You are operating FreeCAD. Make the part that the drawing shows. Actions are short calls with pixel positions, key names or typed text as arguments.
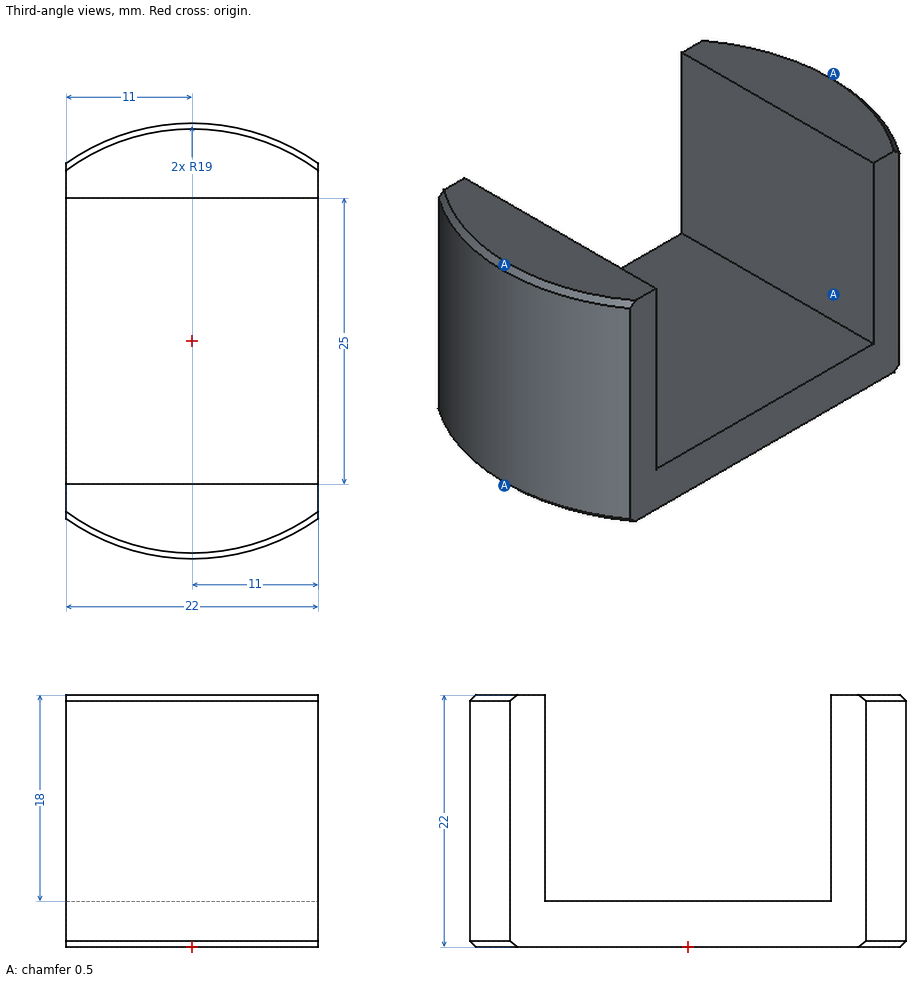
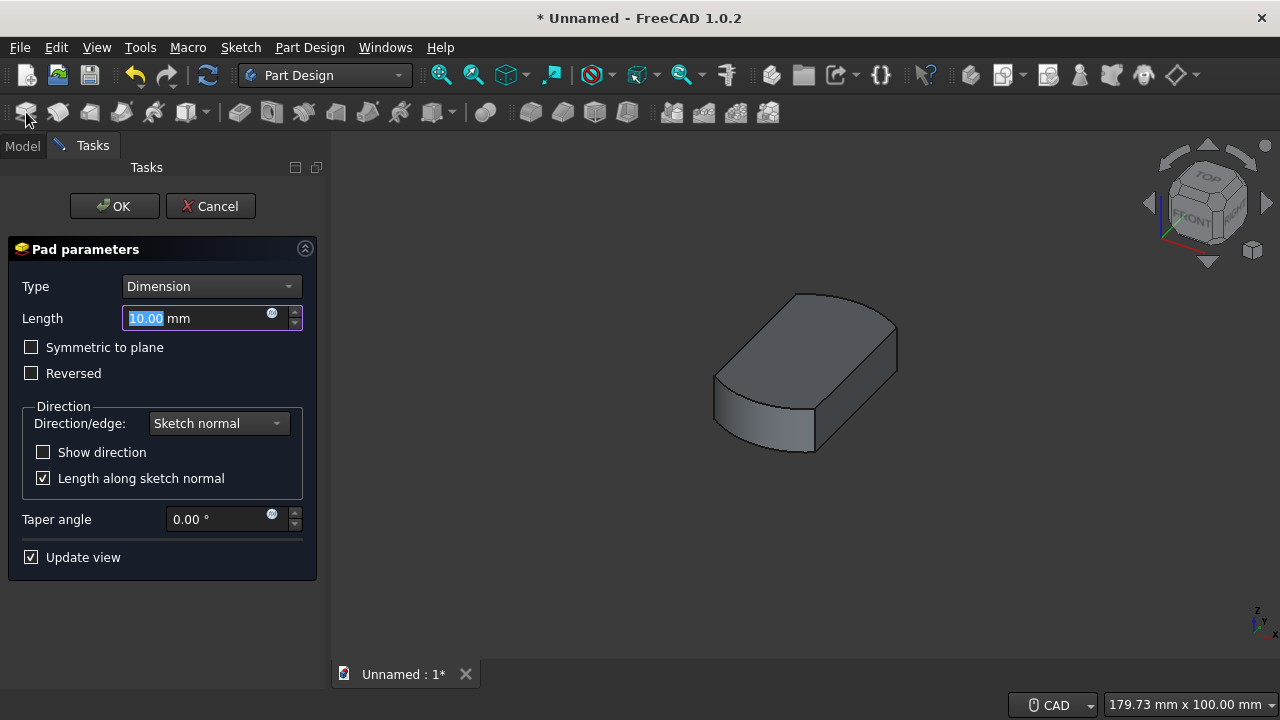
text(22)
key(Tab)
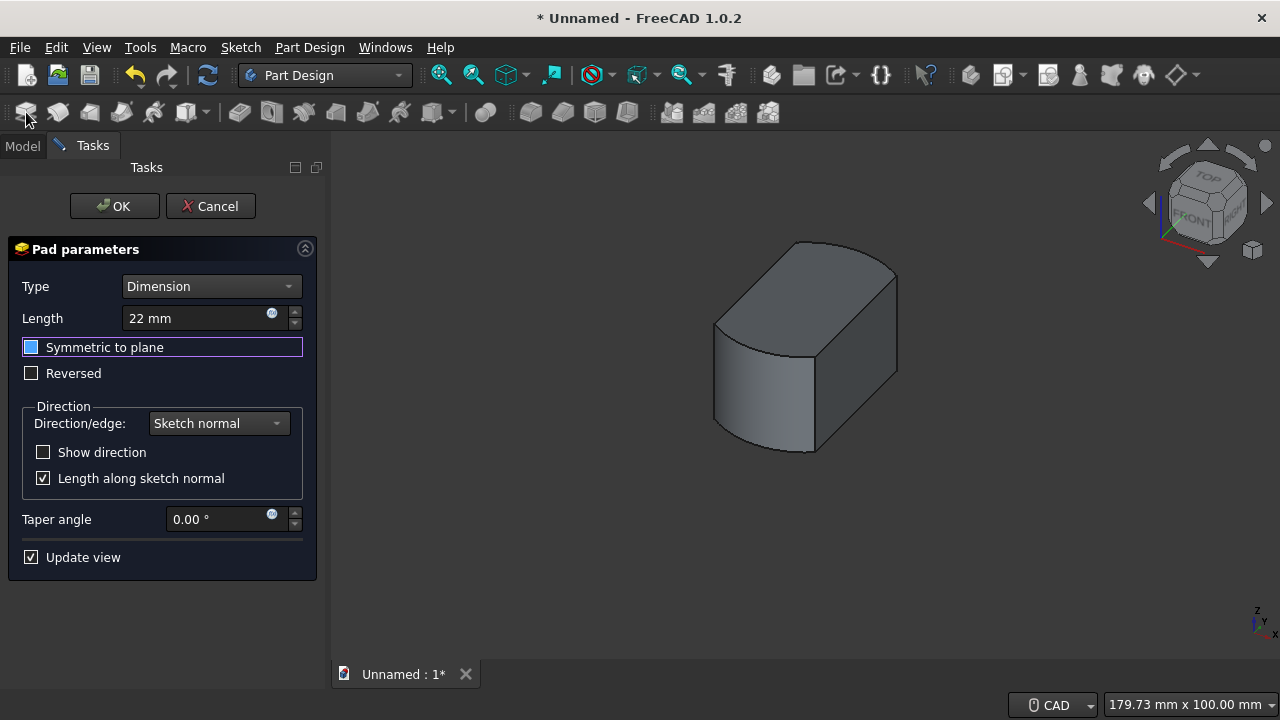
click(115, 206)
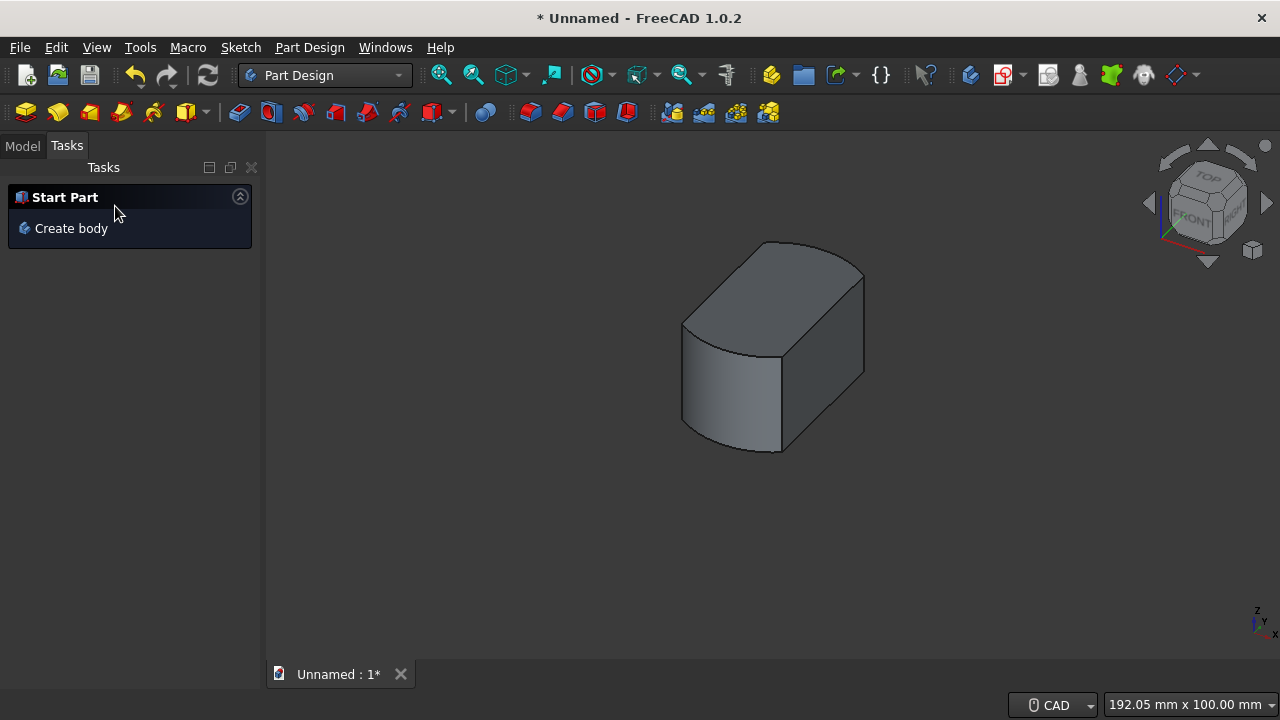
click(442, 76)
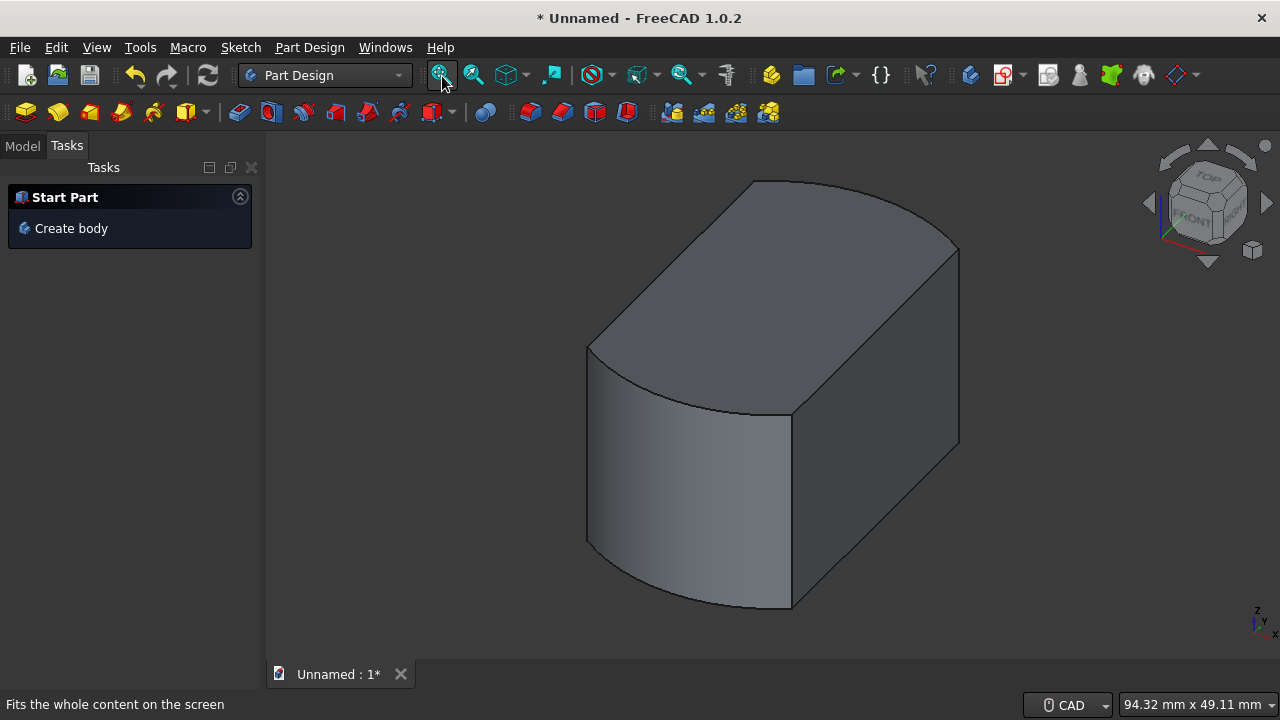
click(802, 268)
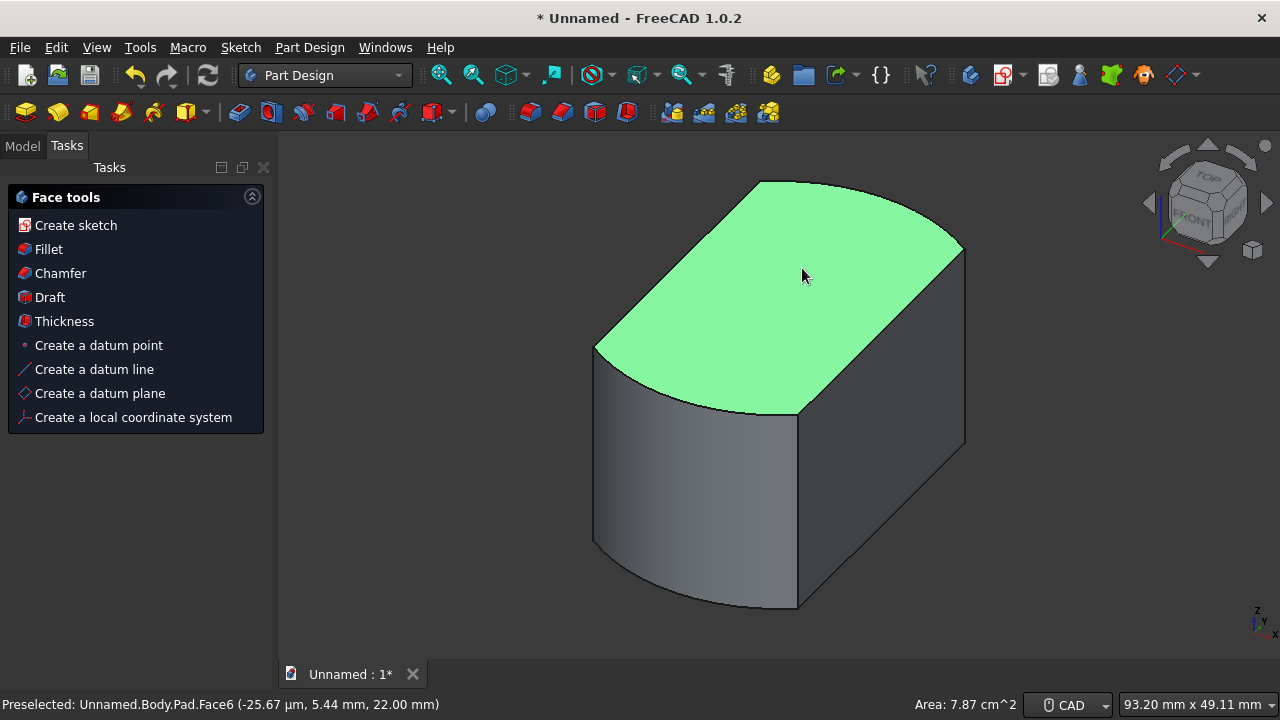
click(1004, 76)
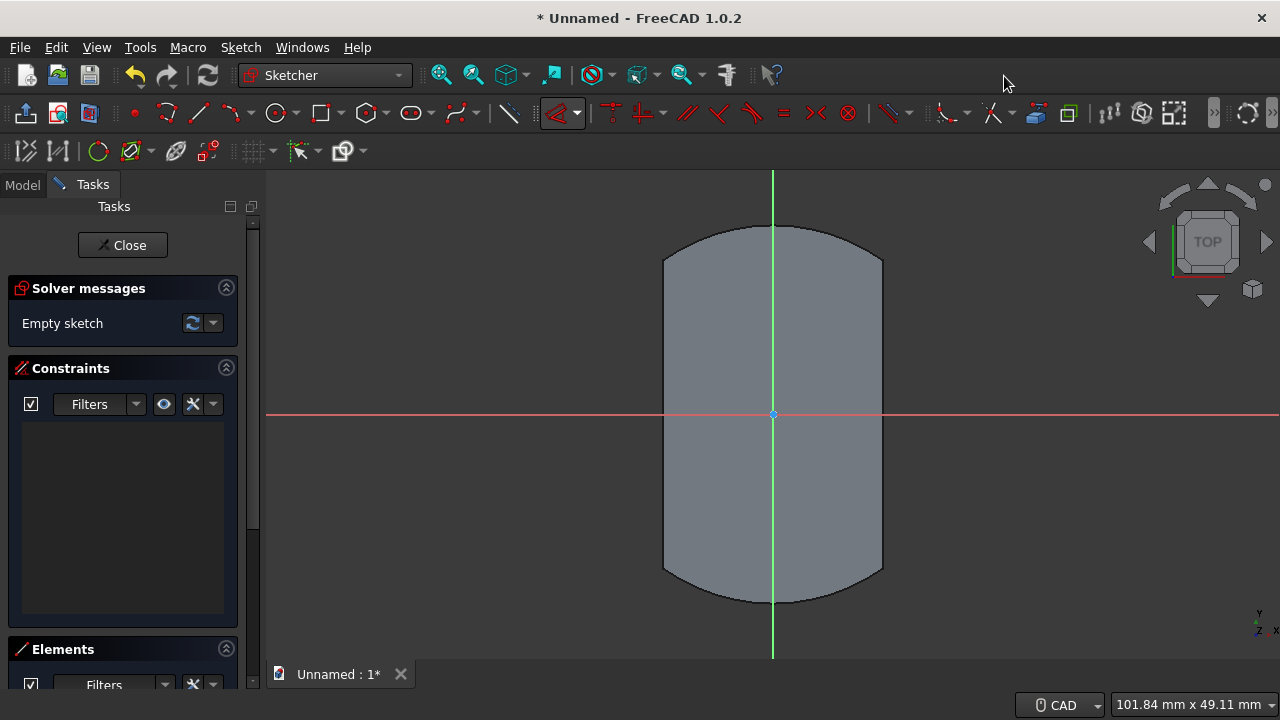
click(344, 114)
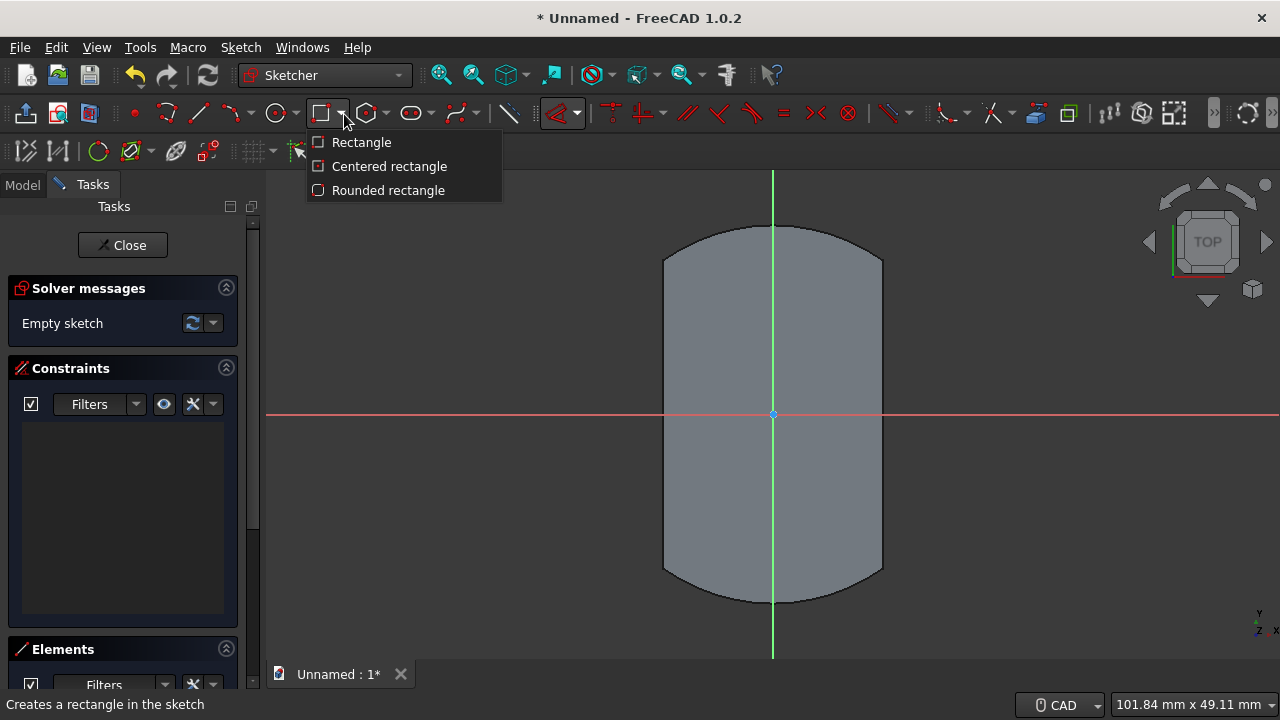
click(404, 166)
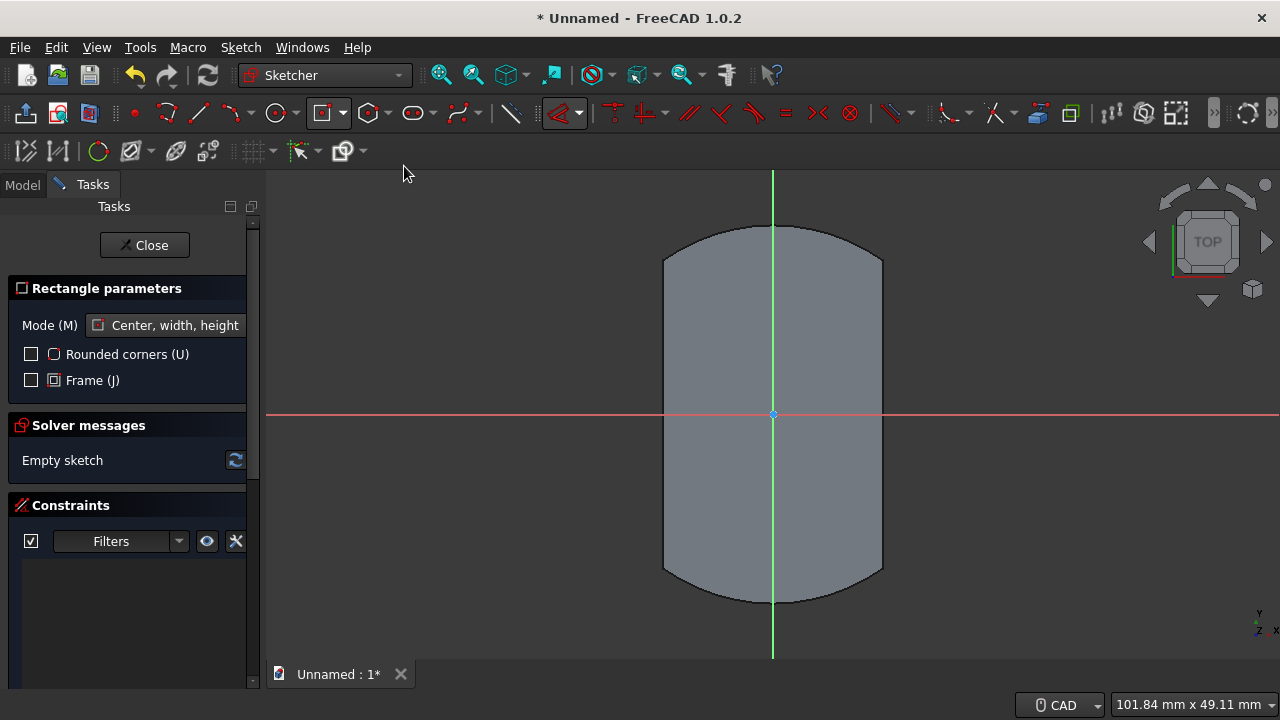
click(773, 414)
move(883, 290)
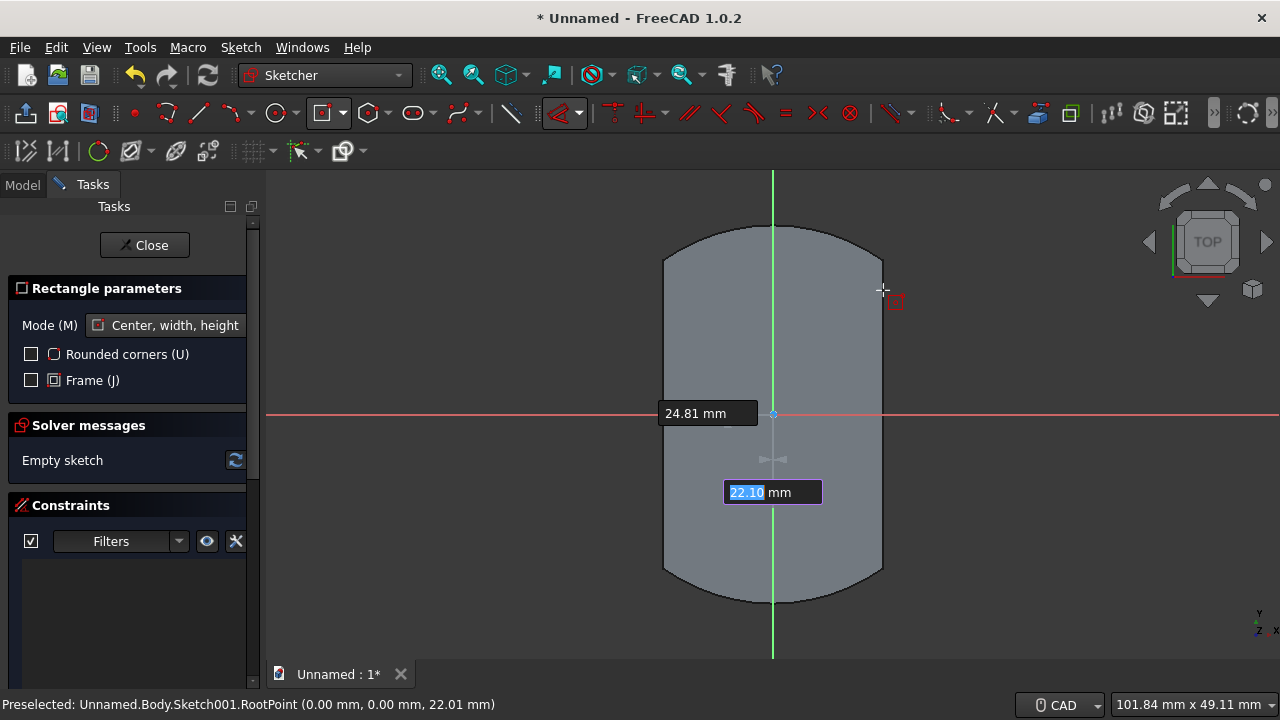
text(22)
key(Tab)
text(25)
key(Return)
key(Escape)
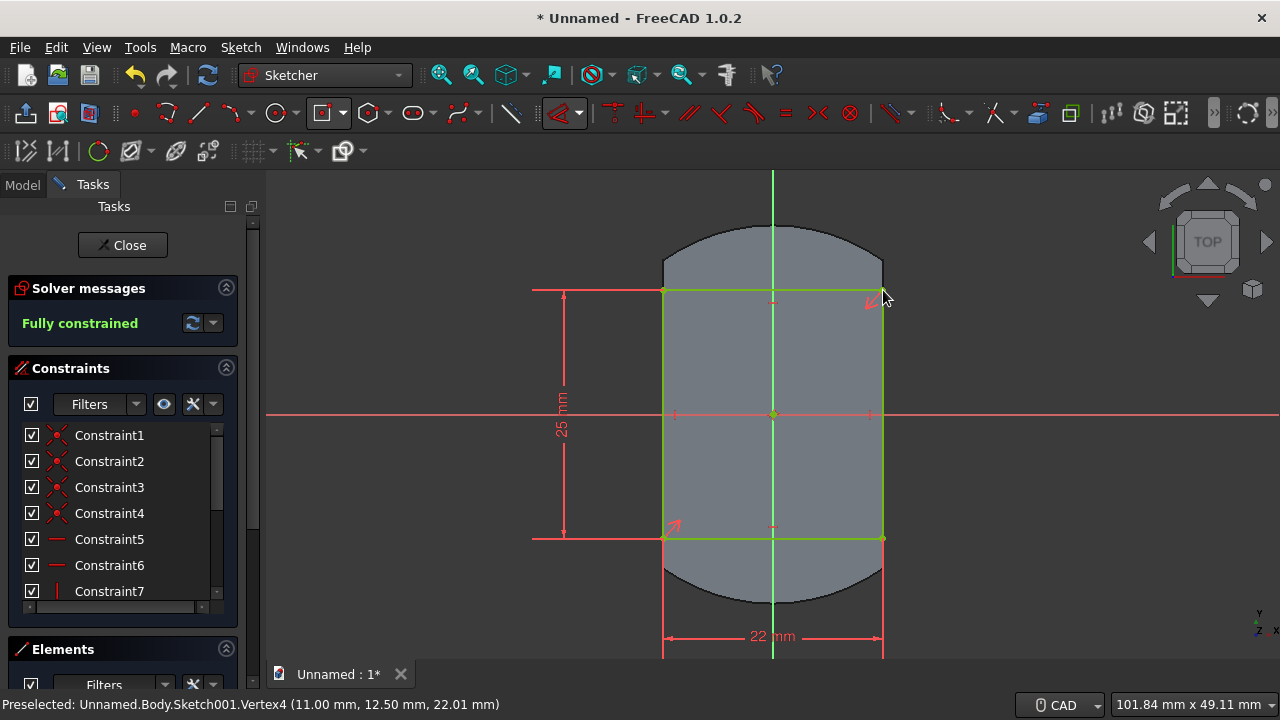
click(123, 245)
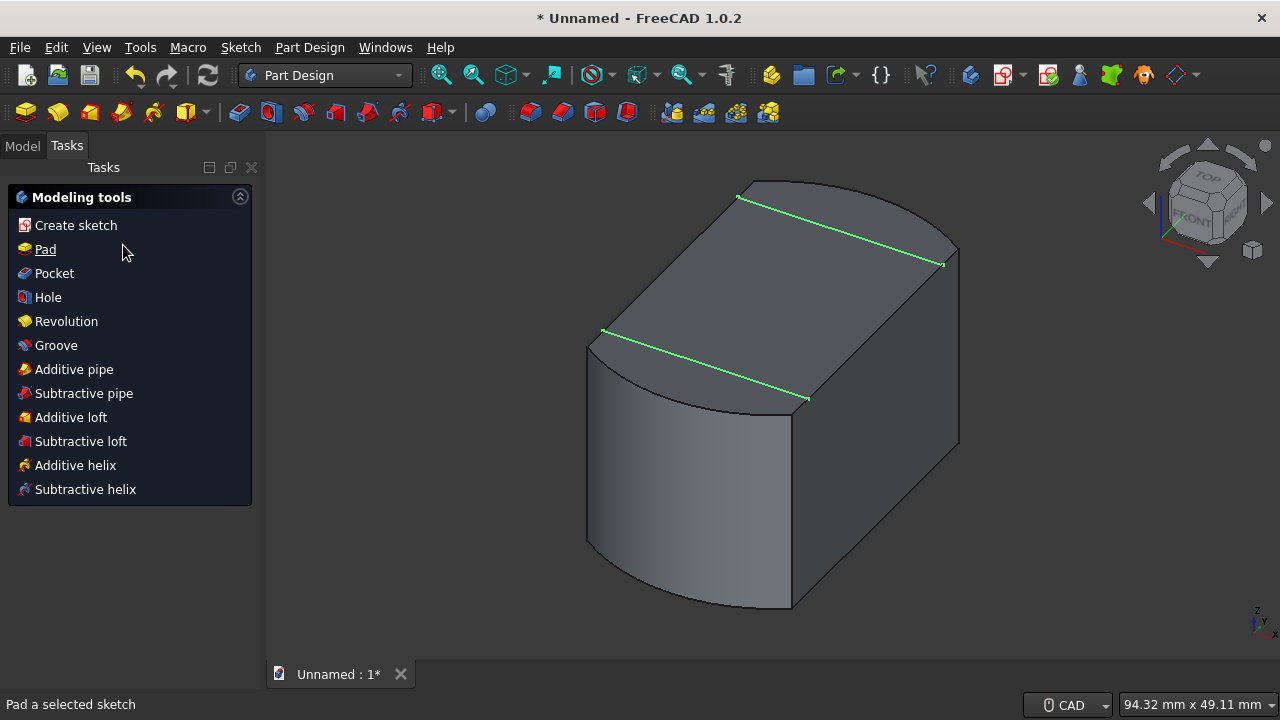
click(240, 112)